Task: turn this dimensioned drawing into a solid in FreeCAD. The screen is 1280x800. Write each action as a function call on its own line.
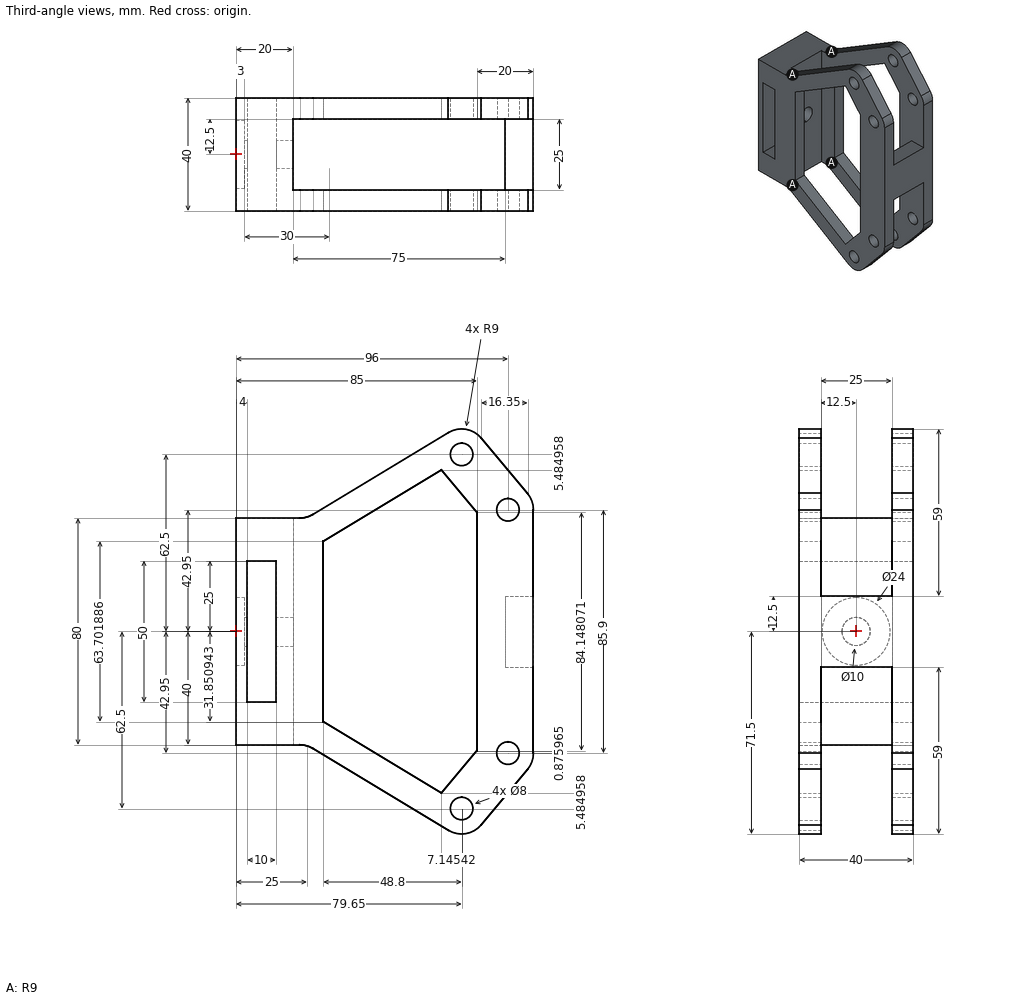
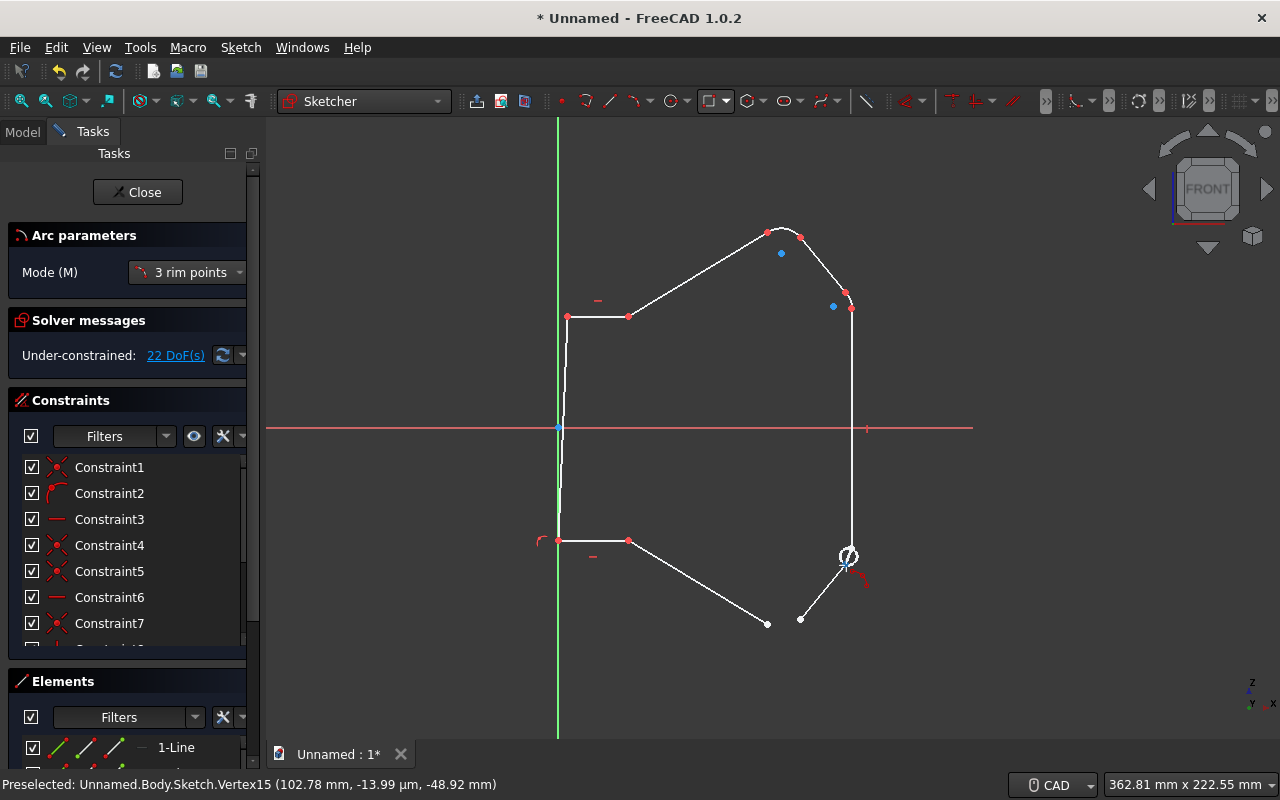
scroll(850, 556, up, 12)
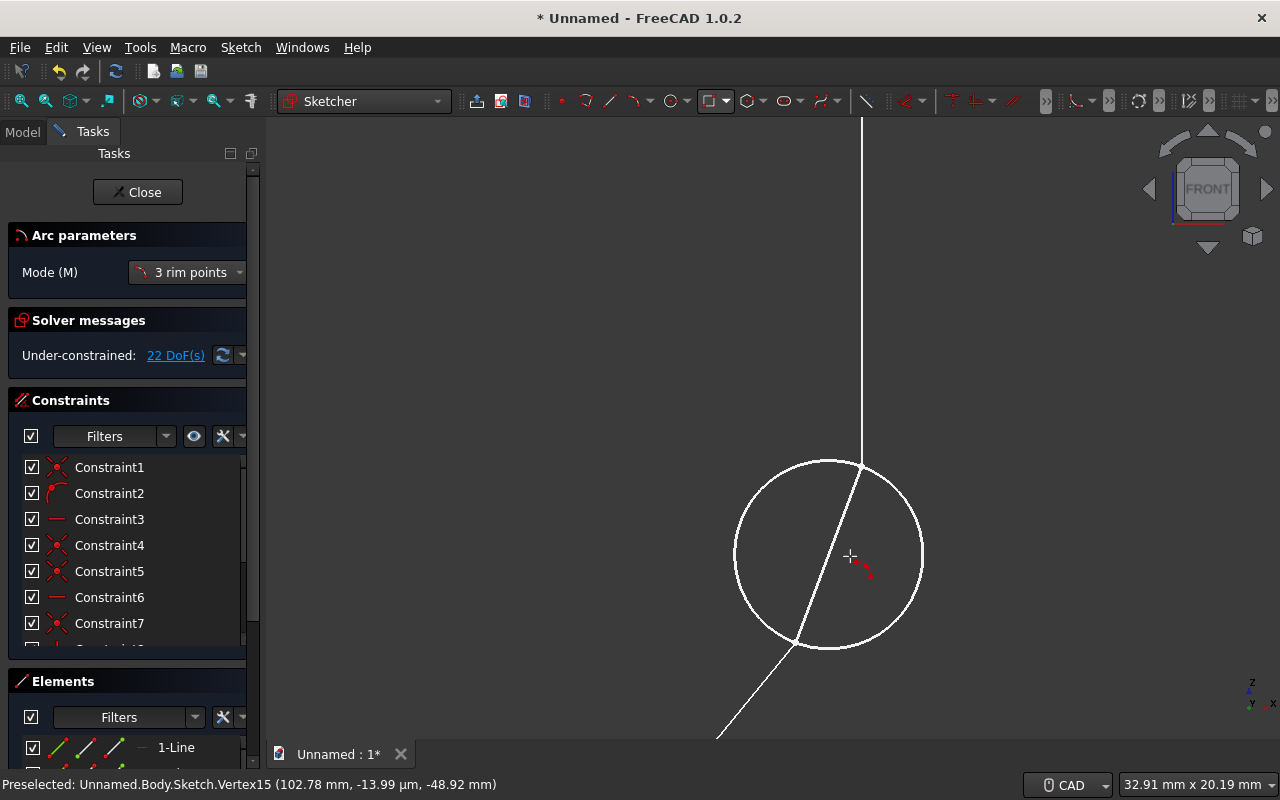
click(847, 554)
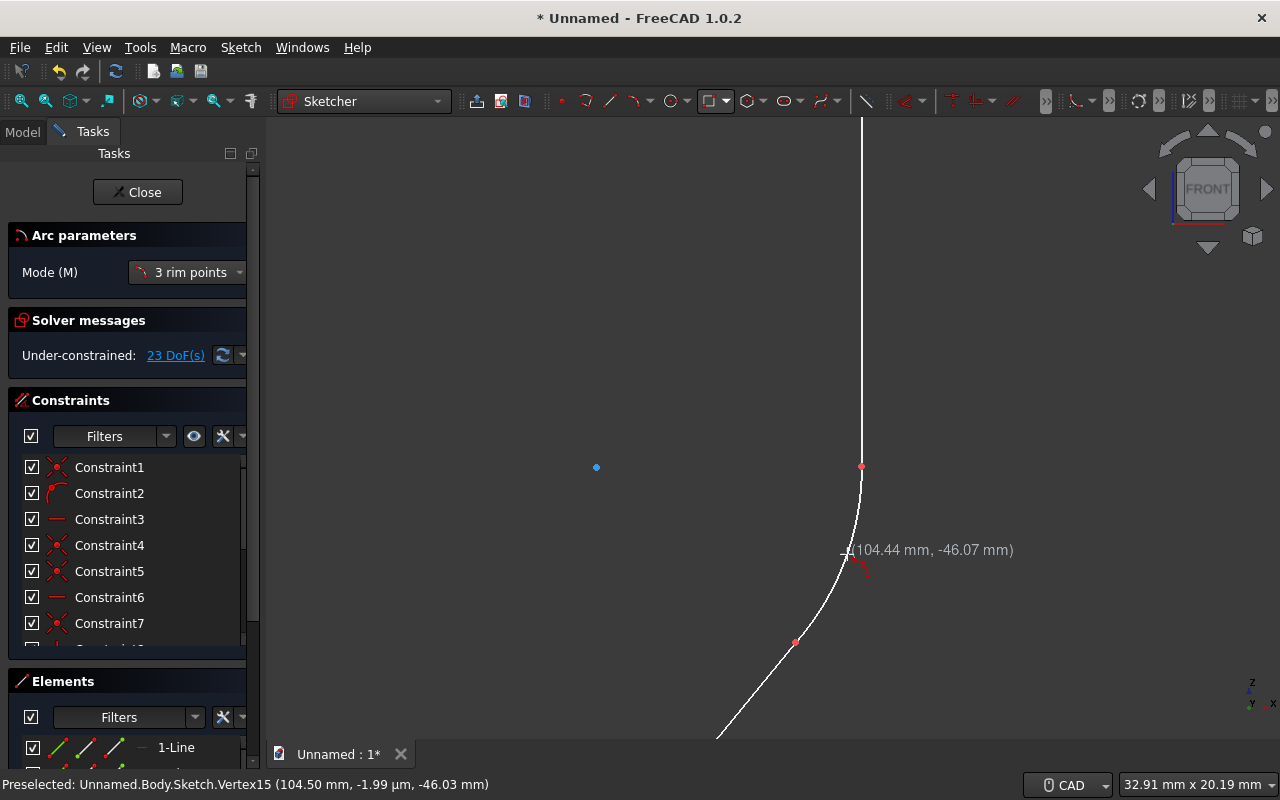
scroll(850, 557, down, 12)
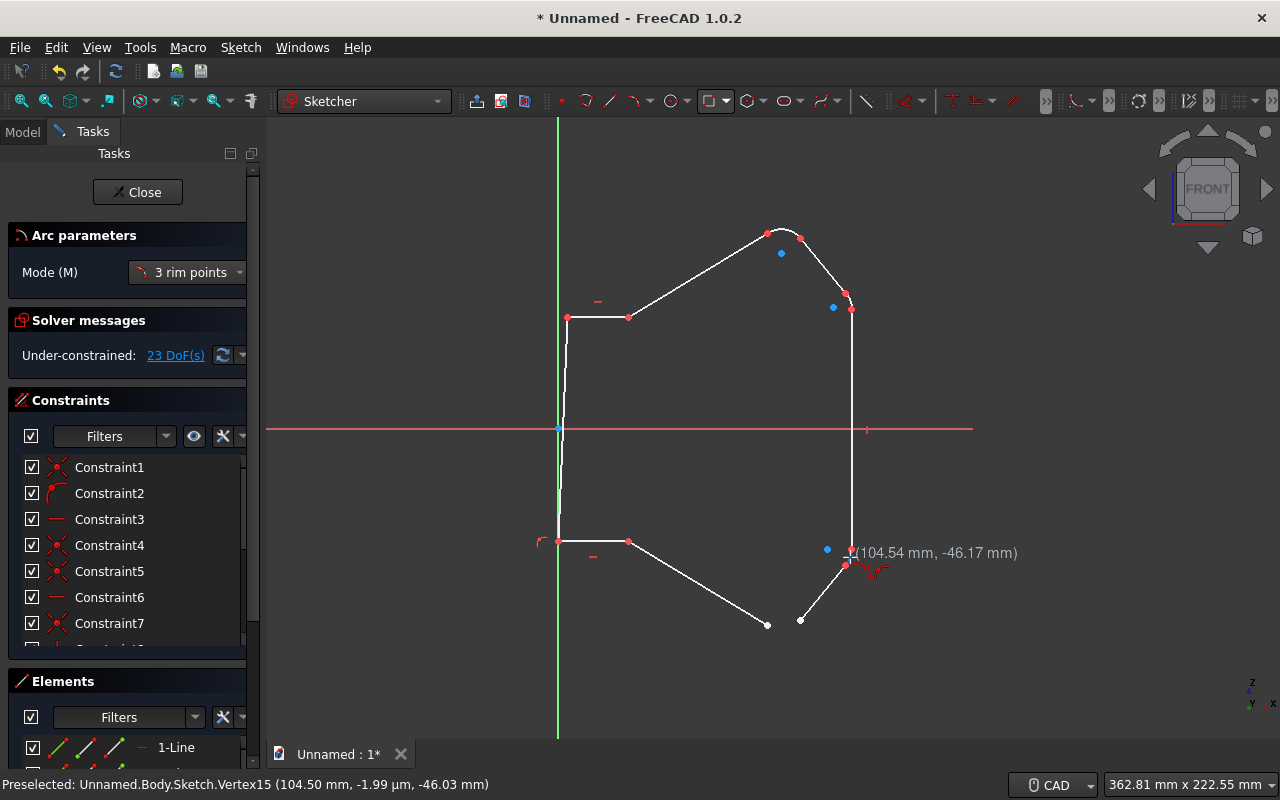
click(801, 620)
click(768, 625)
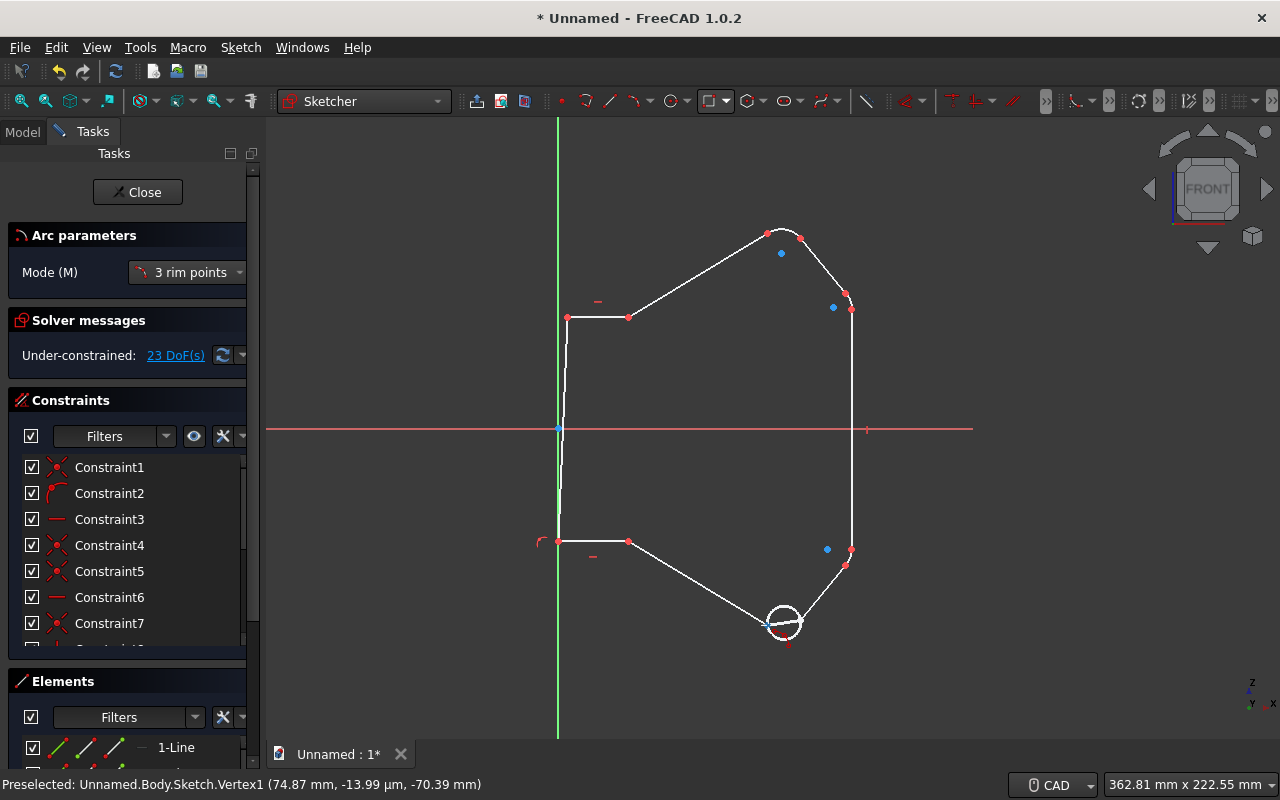
scroll(785, 628, up, 5)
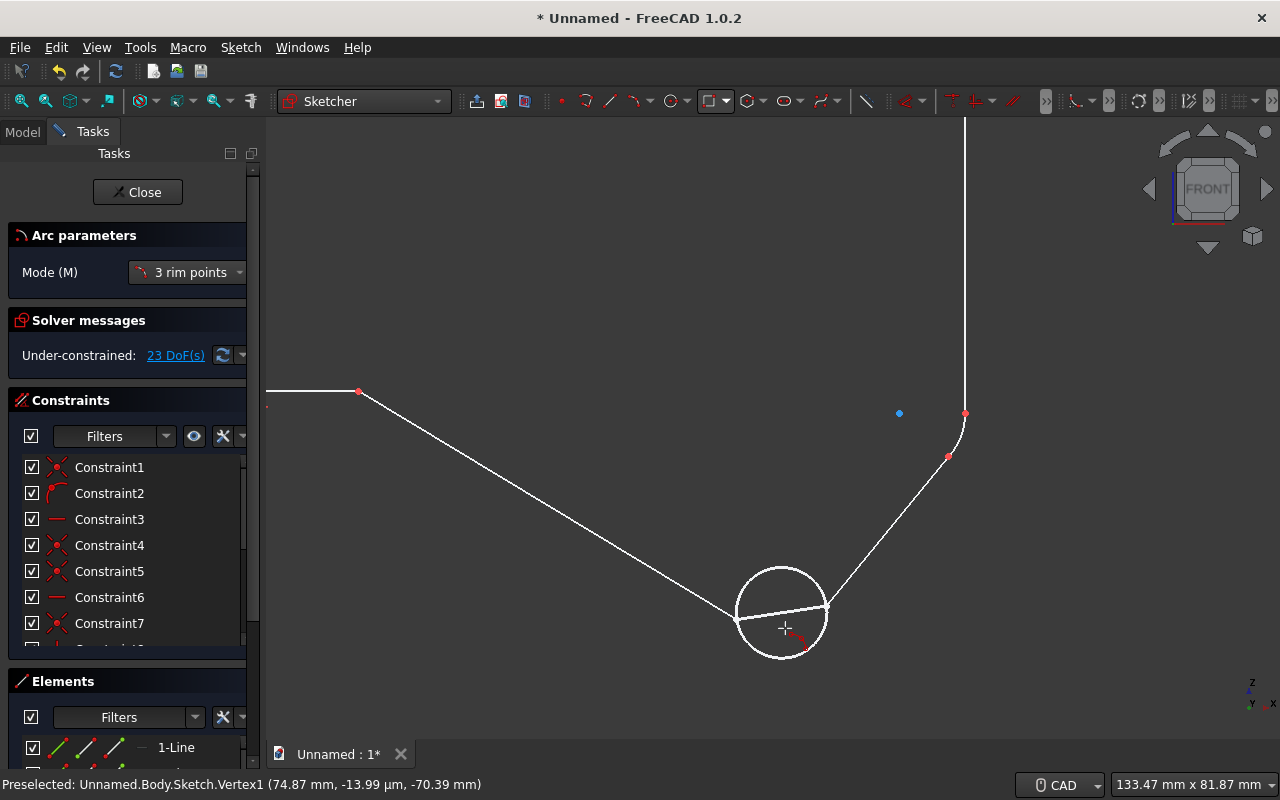
click(784, 627)
key(Escape)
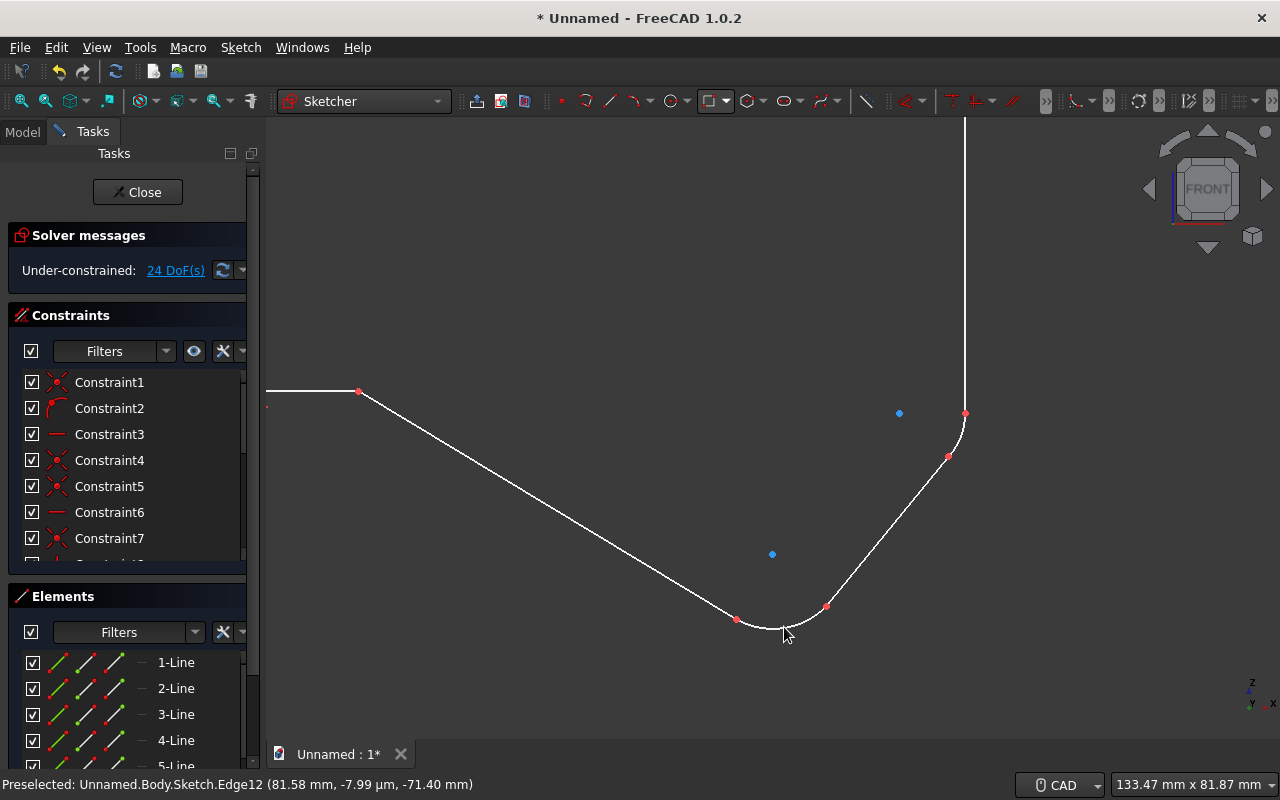
click(623, 551)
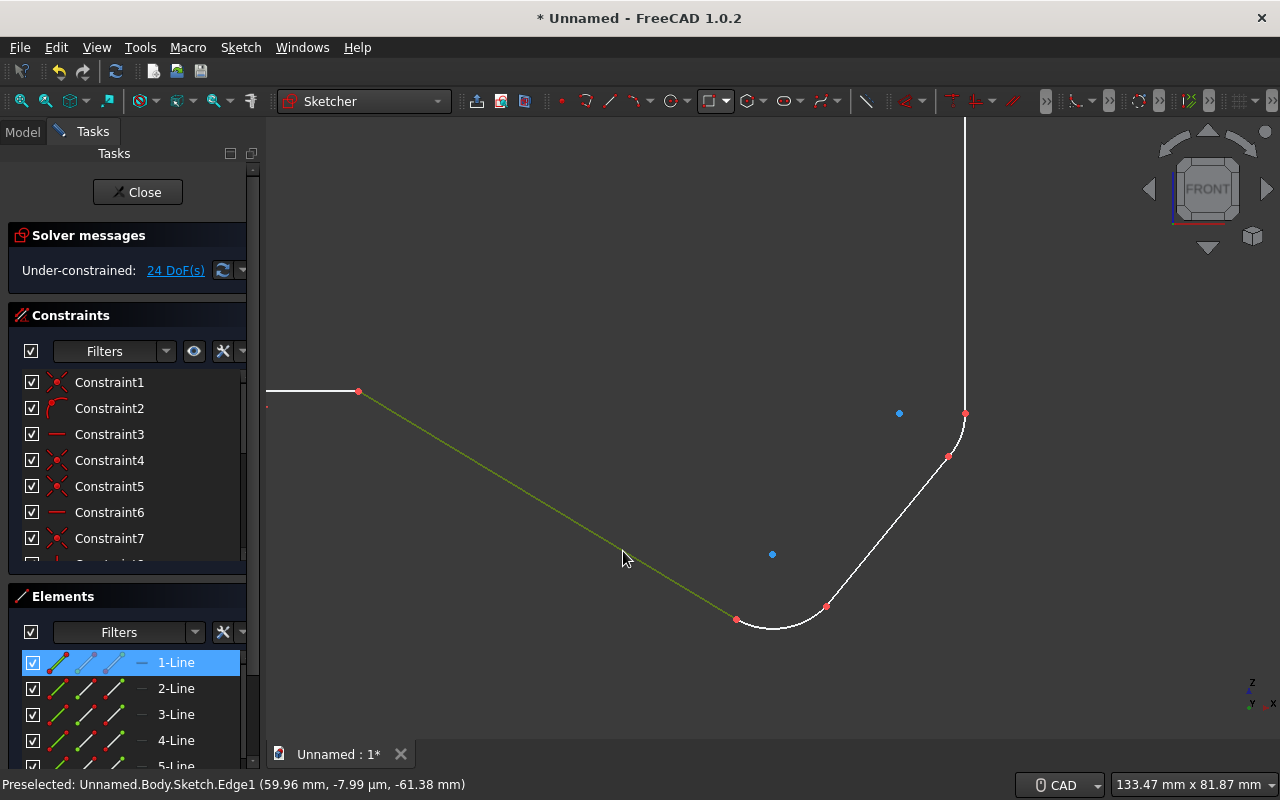
click(765, 628)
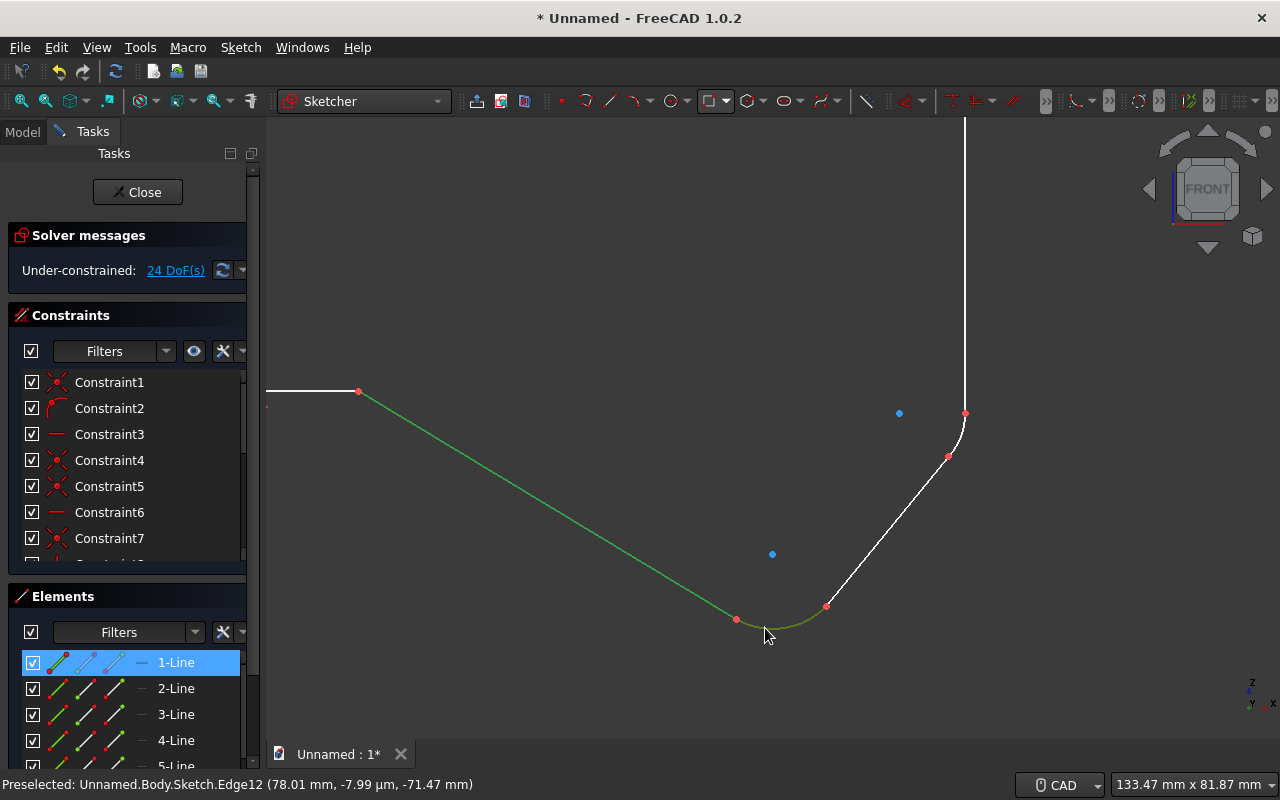
key(t)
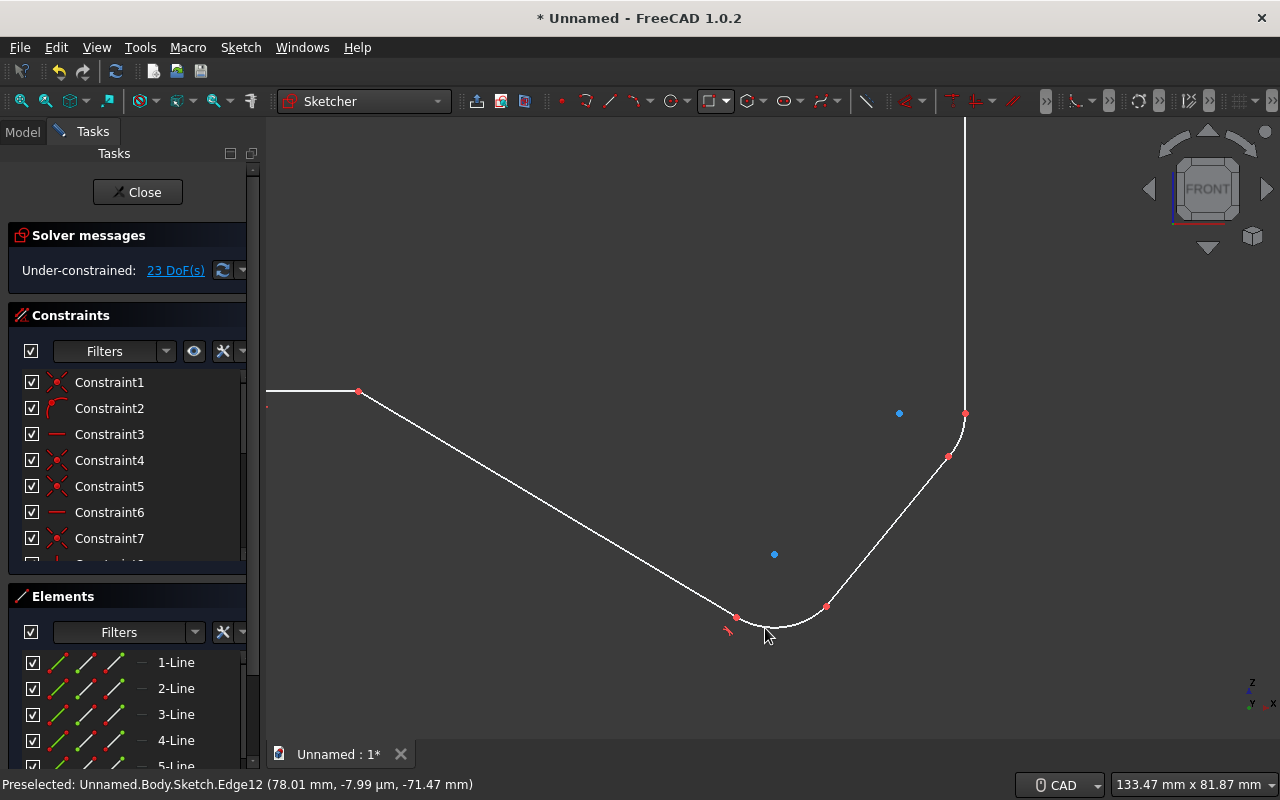
scroll(785, 628, down, 5)